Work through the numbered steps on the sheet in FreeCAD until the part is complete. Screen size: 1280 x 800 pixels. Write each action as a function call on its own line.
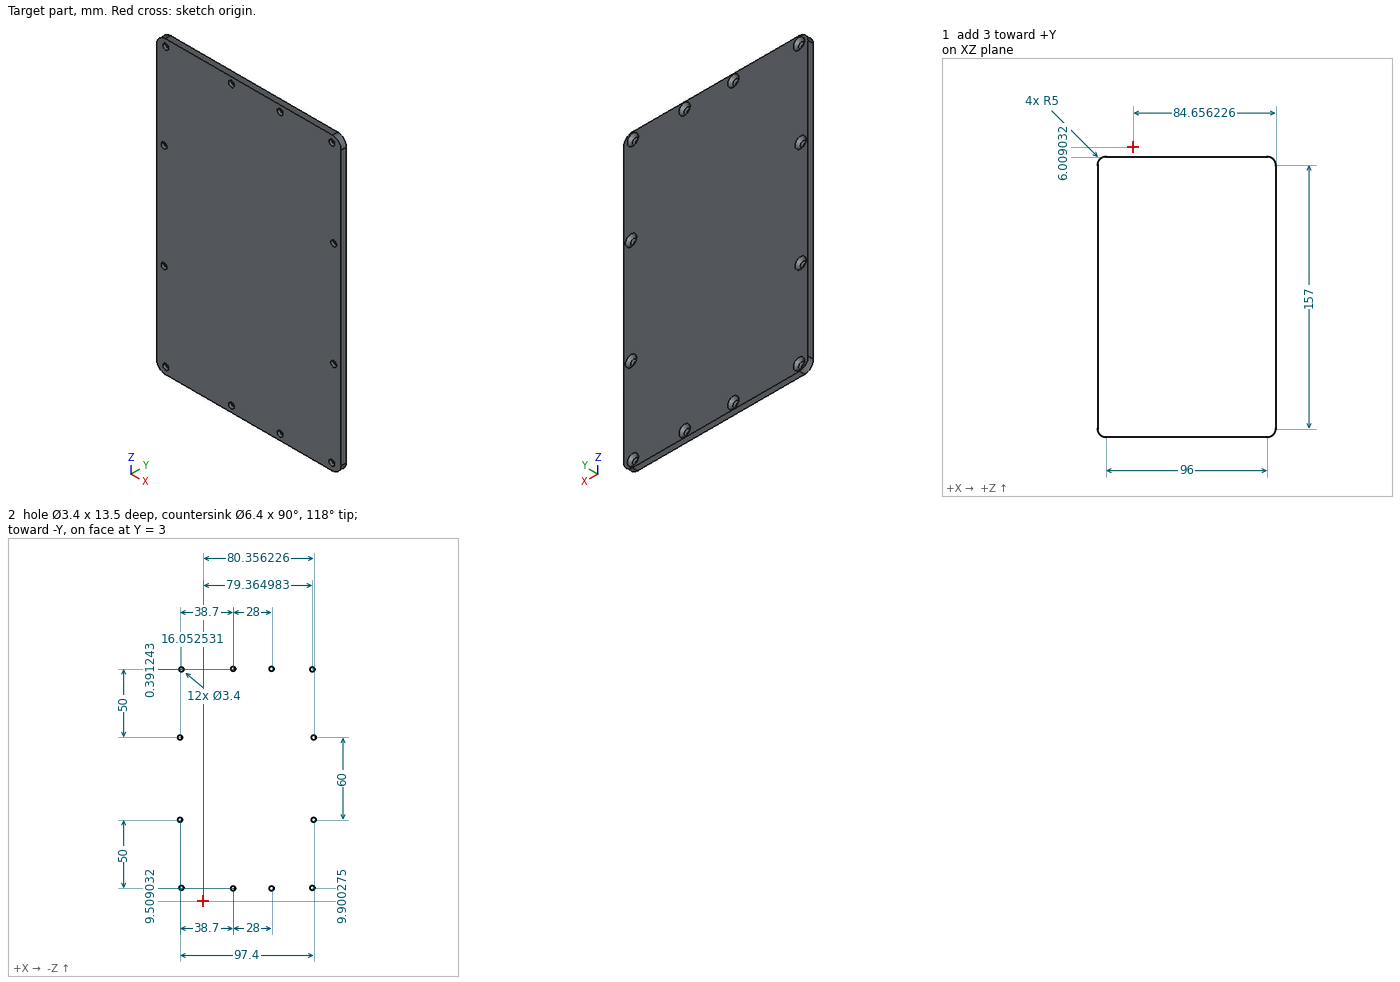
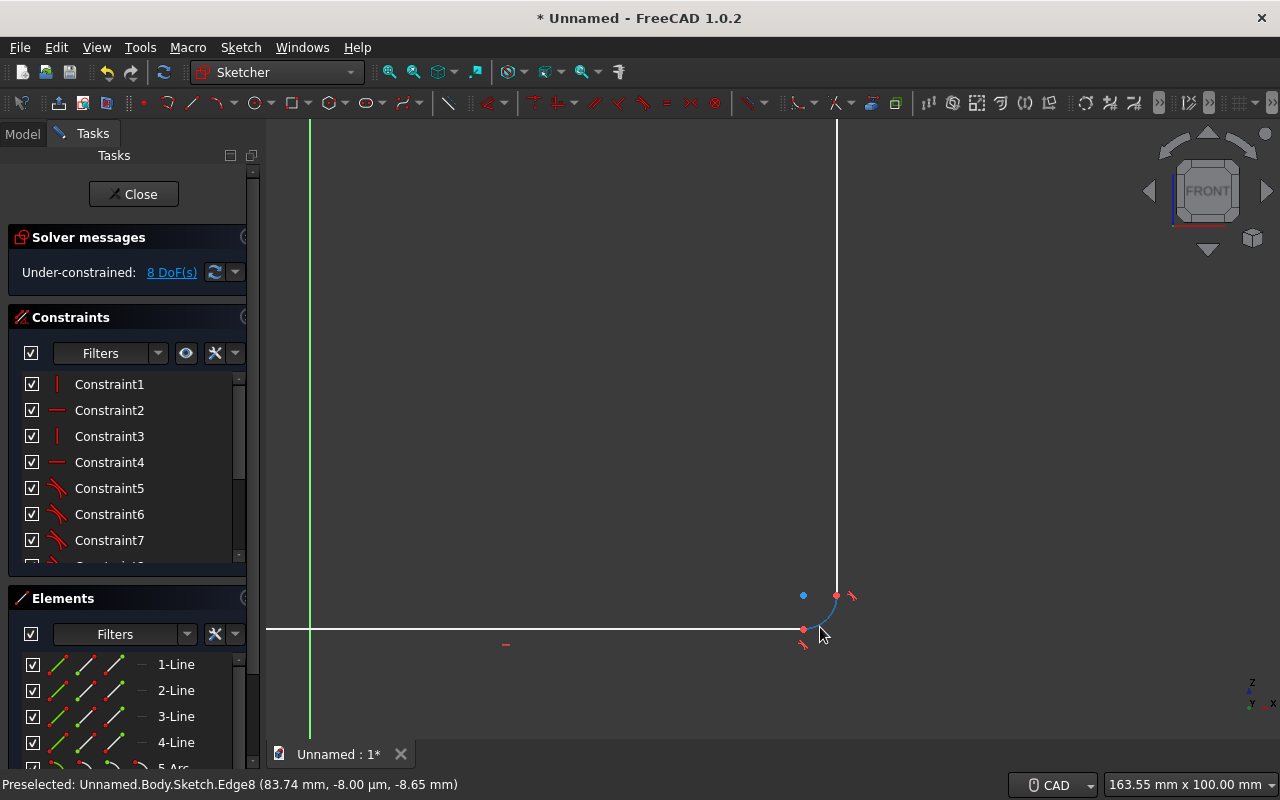
click(818, 625)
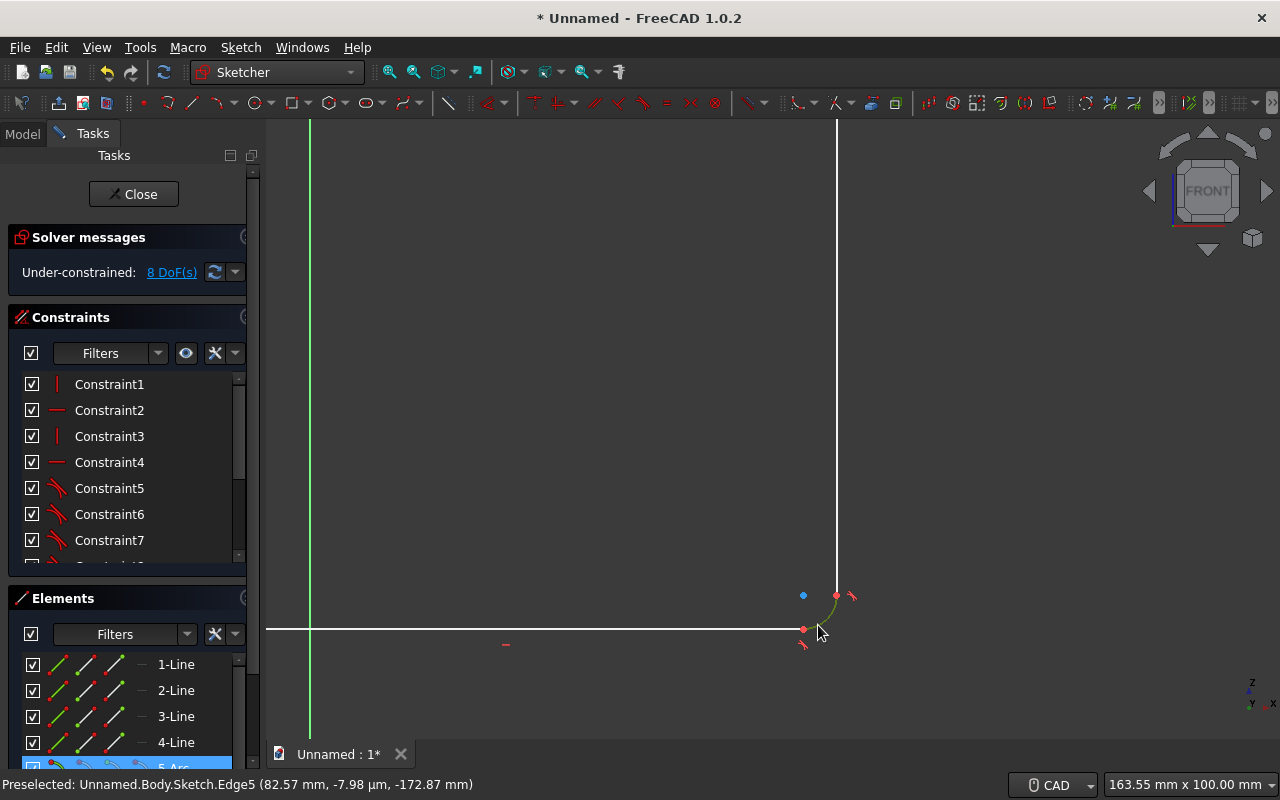
scroll(820, 628, down, 5)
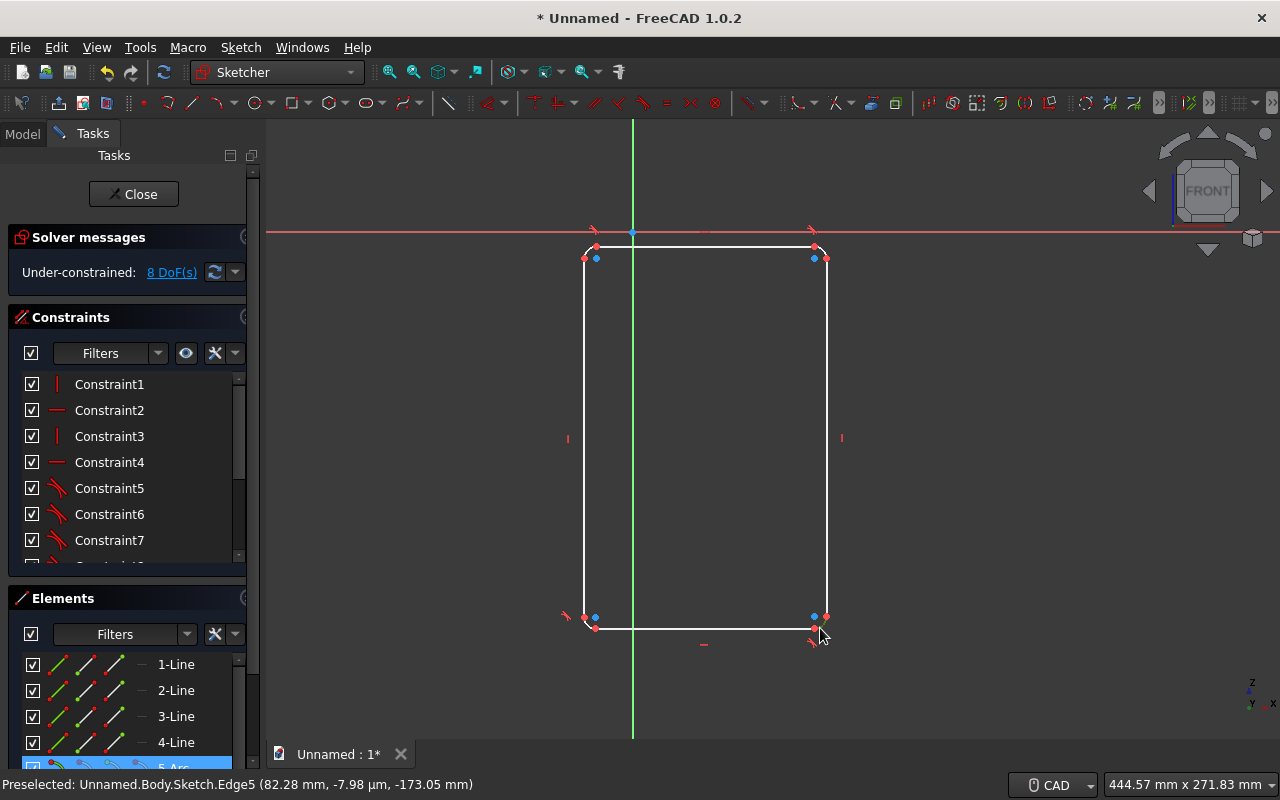
scroll(586, 623, up, 5)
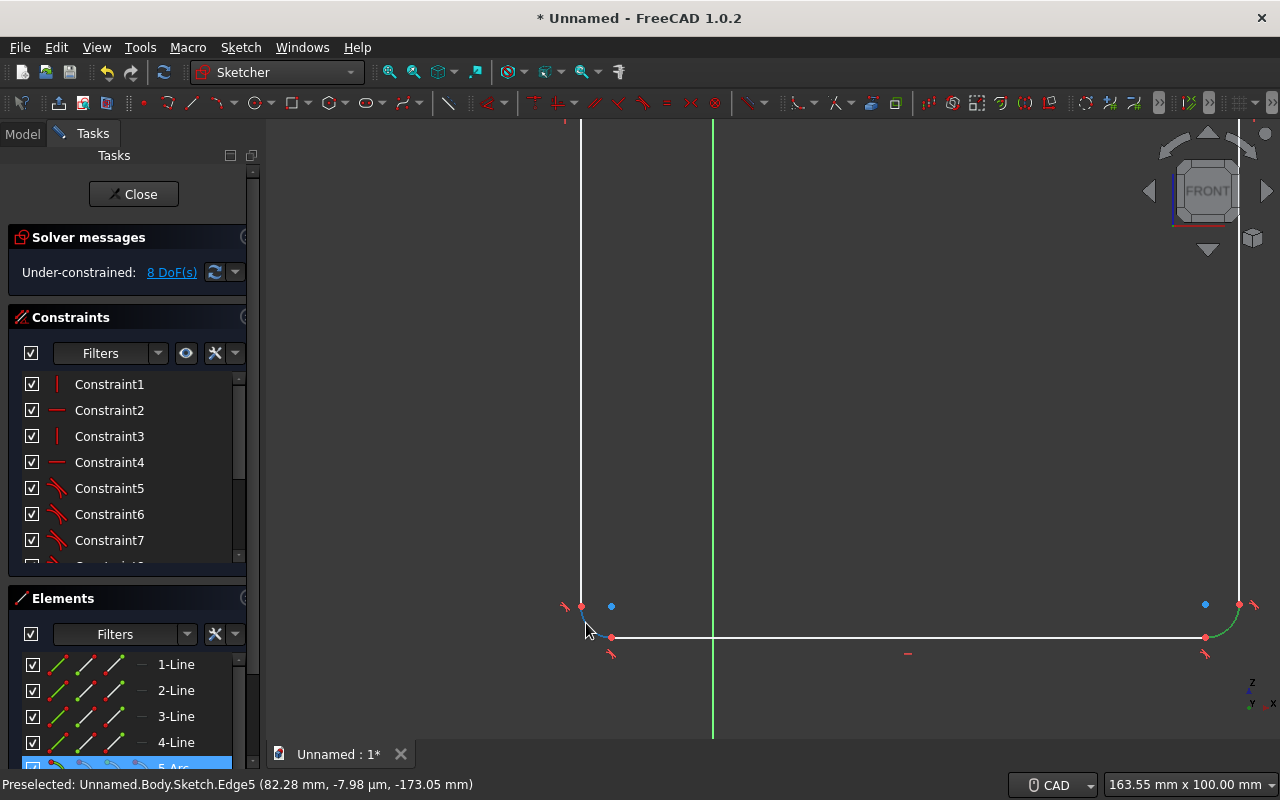
click(584, 621)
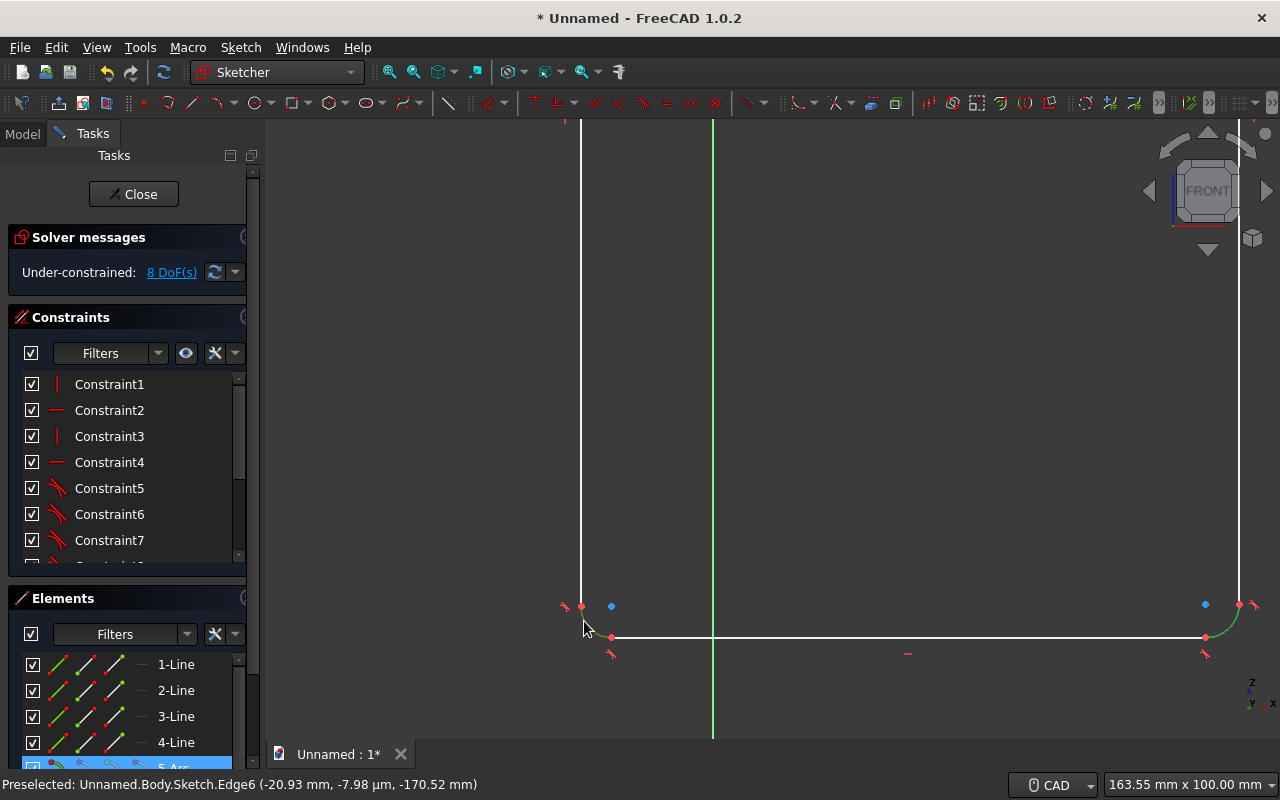
scroll(586, 623, down, 5)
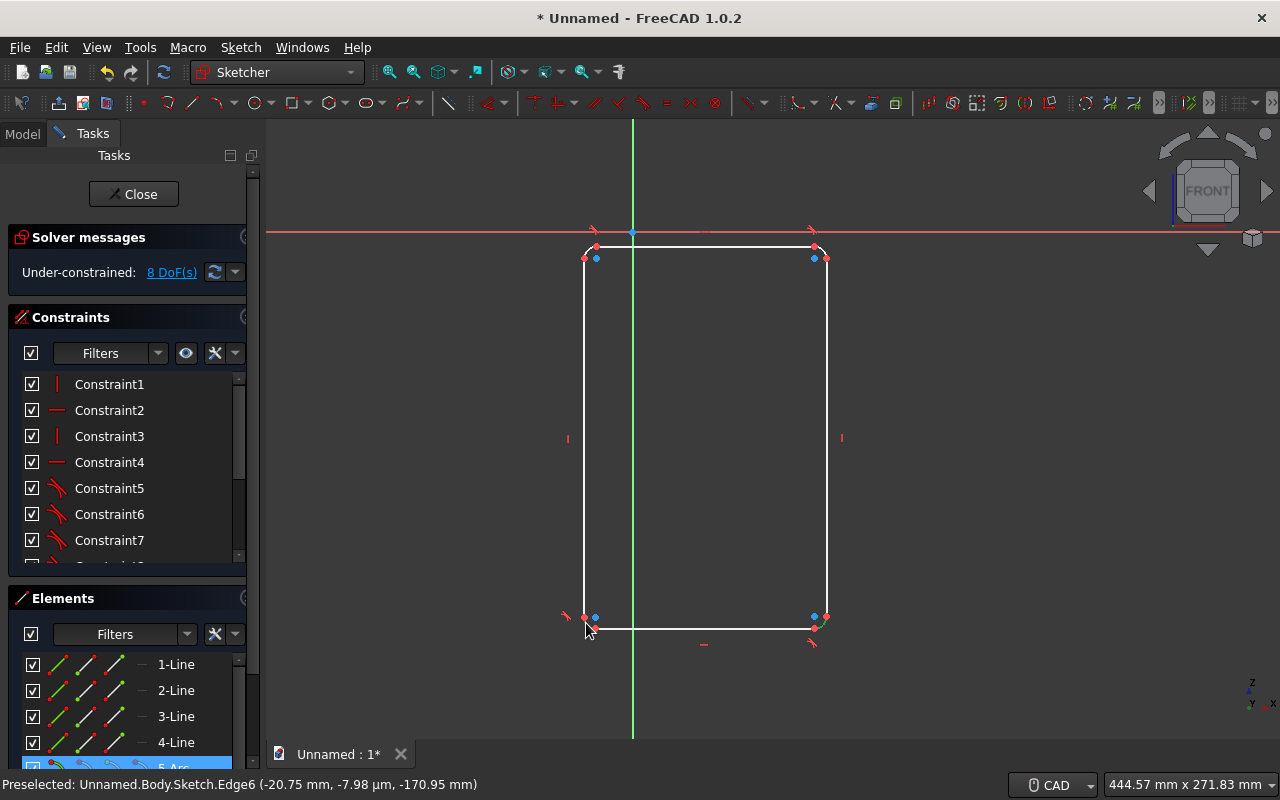
scroll(591, 248, up, 5)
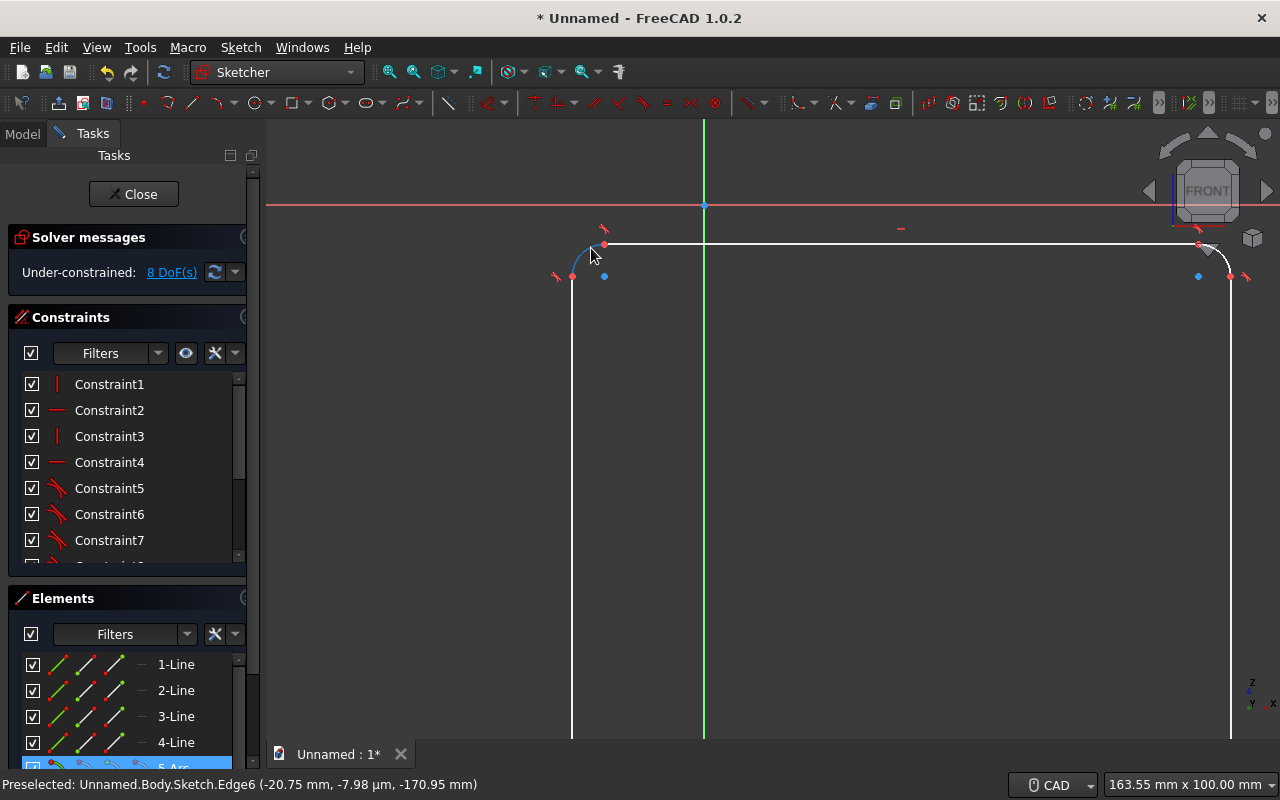
click(590, 248)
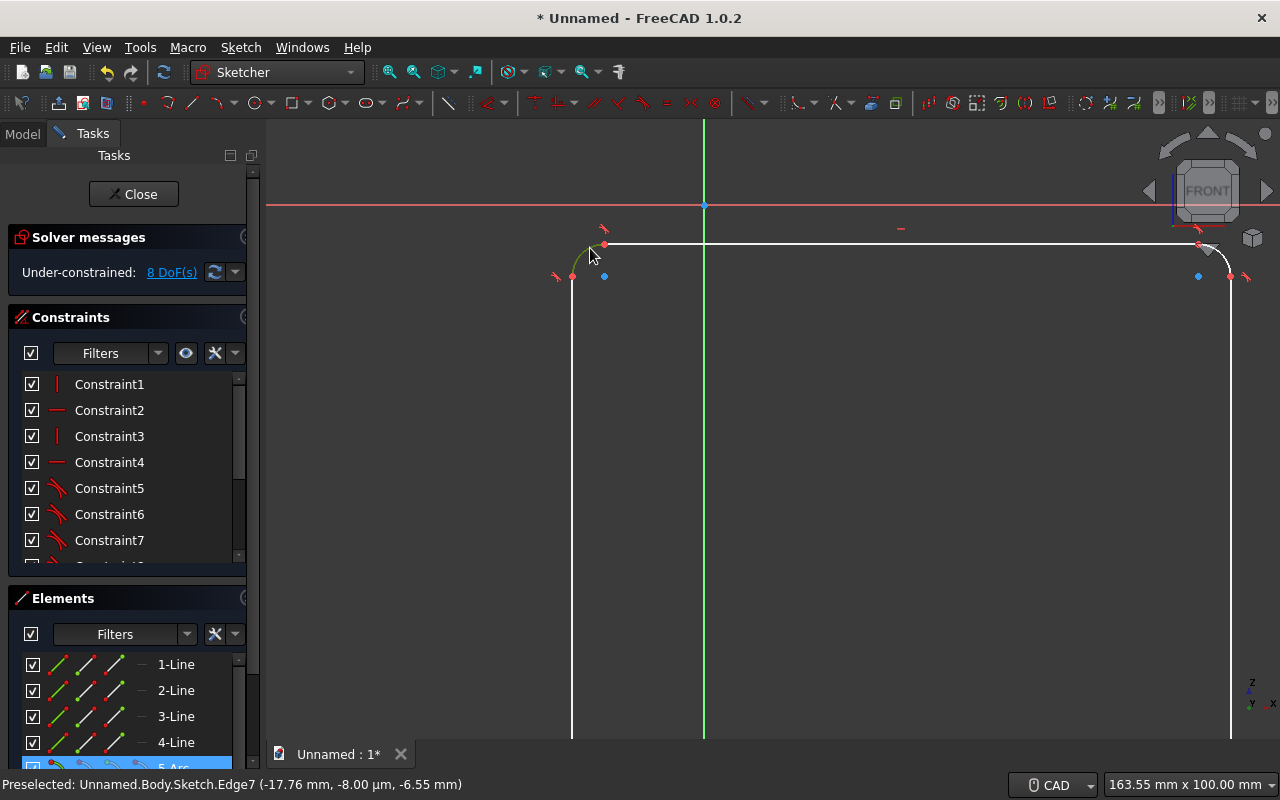
scroll(591, 247, down, 5)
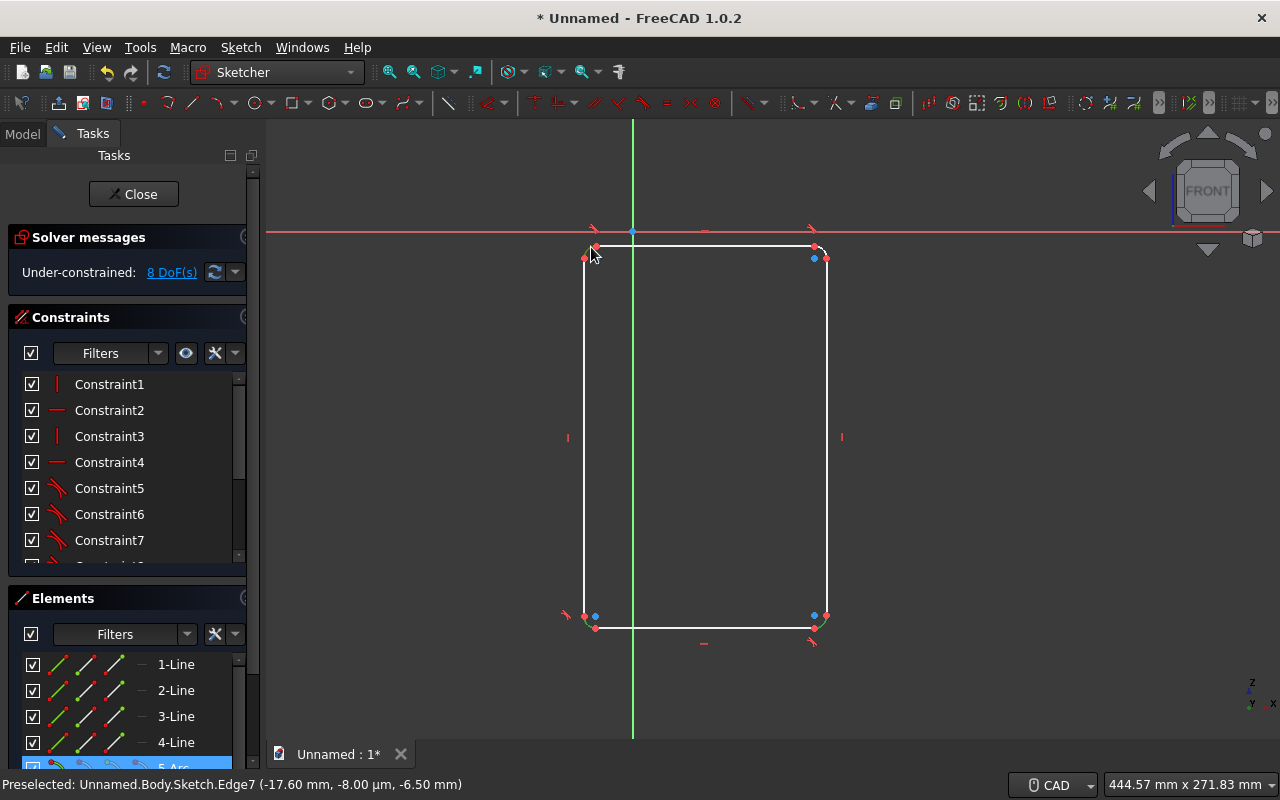
scroll(825, 253, up, 5)